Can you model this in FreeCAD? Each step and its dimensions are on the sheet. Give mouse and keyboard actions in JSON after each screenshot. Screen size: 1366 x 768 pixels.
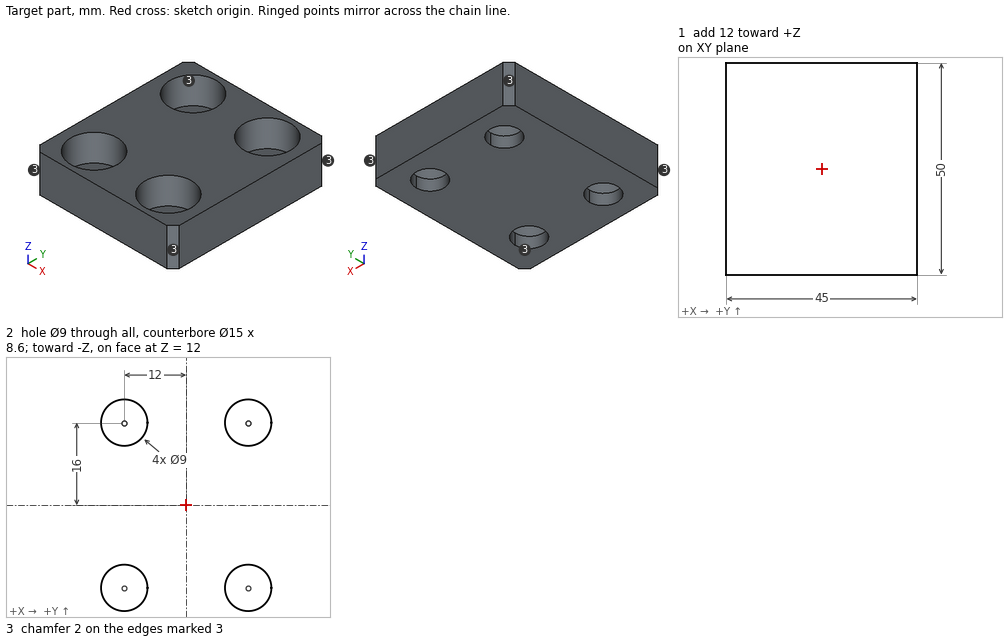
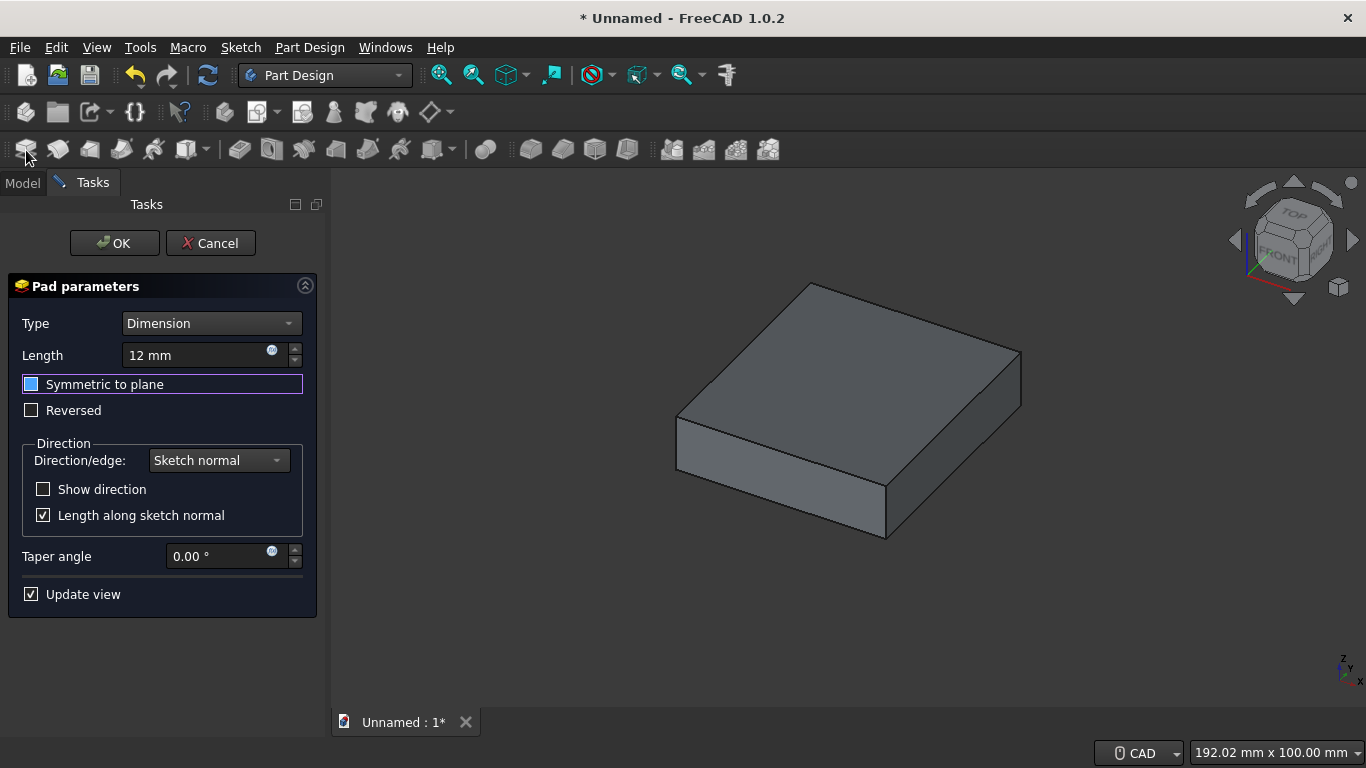
{"action": "left_click", "coordinate": [115, 243]}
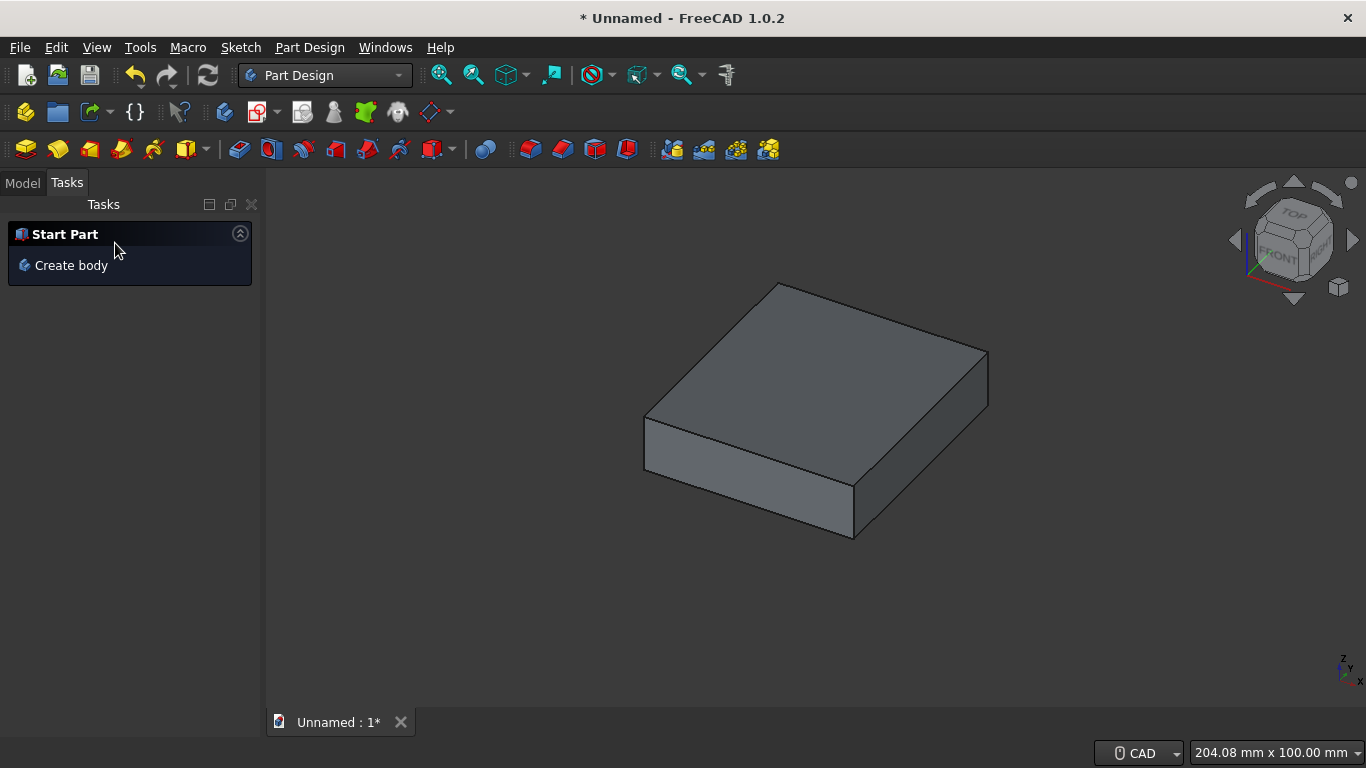
{"action": "left_click", "coordinate": [816, 384]}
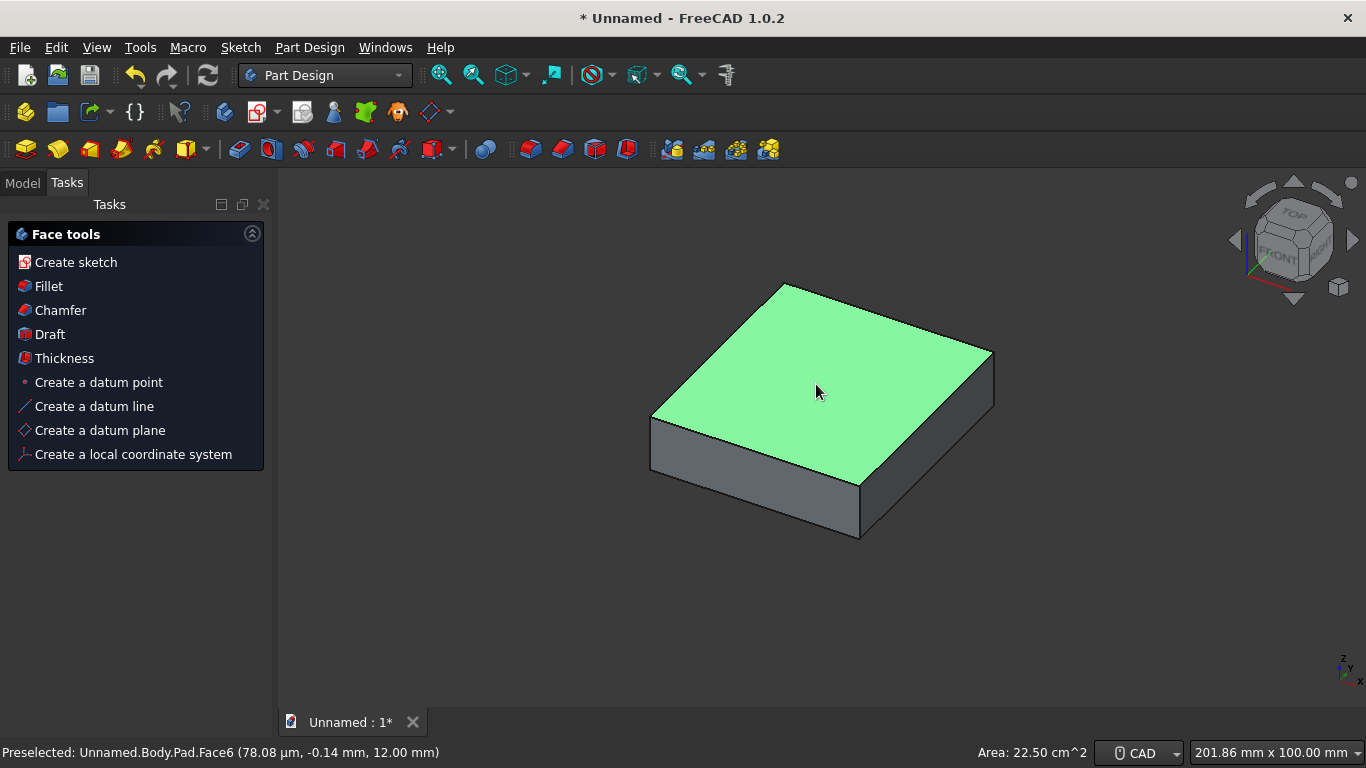
{"action": "left_click", "coordinate": [258, 112]}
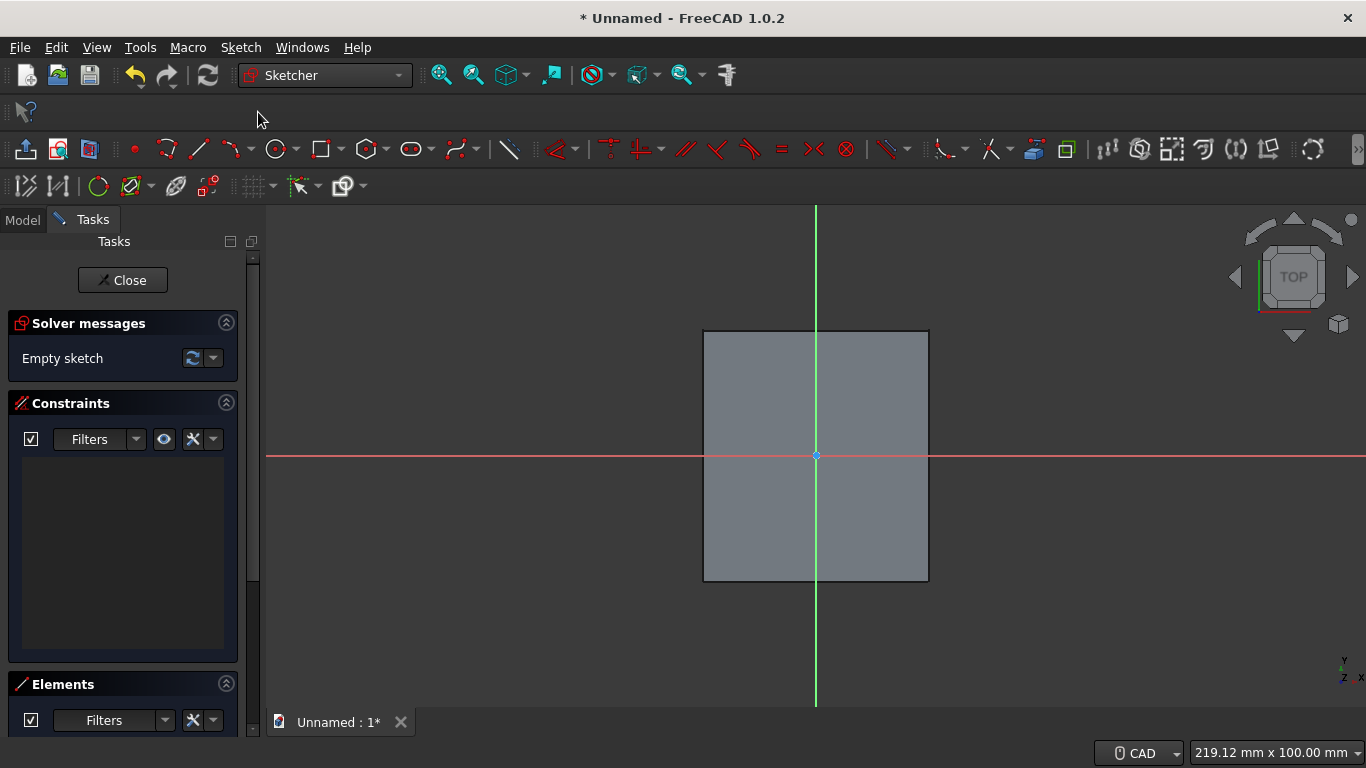
{"action": "scroll", "coordinate": [955, 456], "scroll_direction": "up", "scroll_amount": 2}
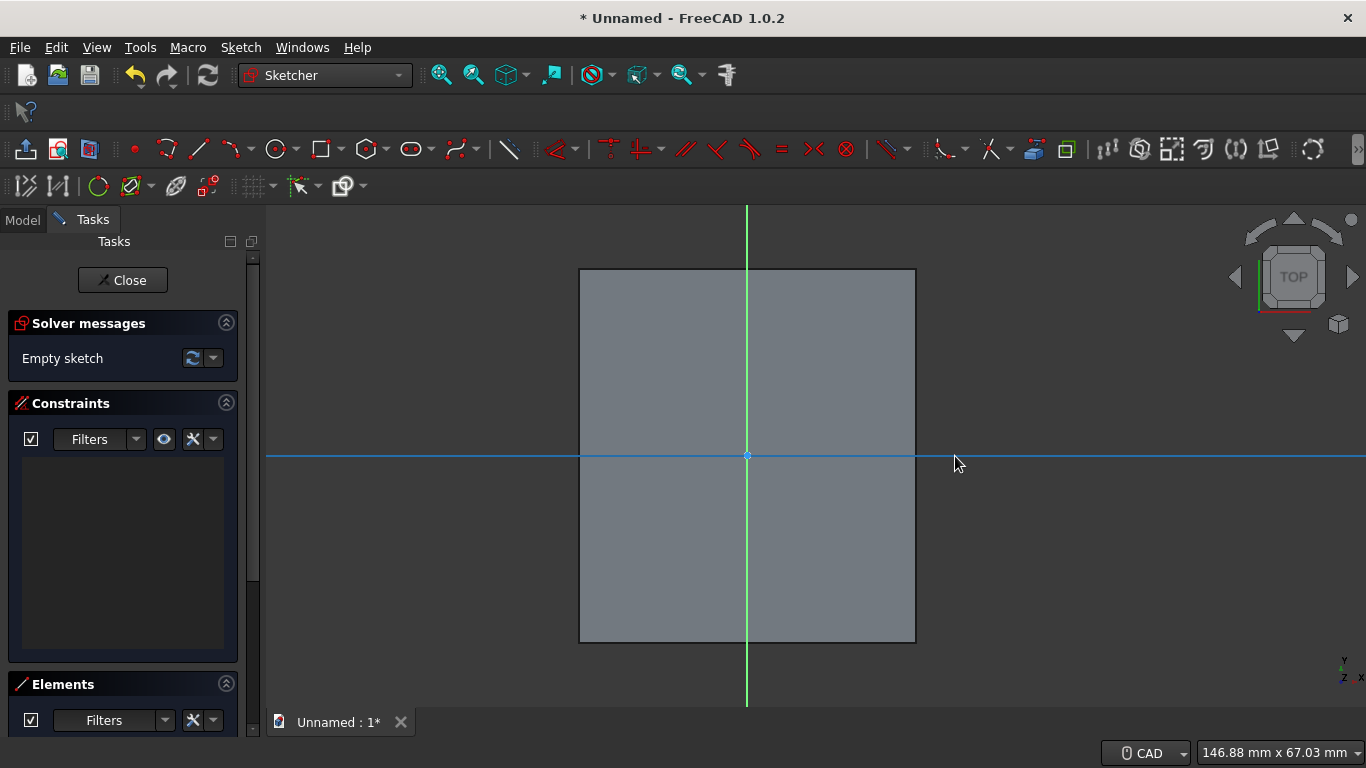
{"action": "left_click", "coordinate": [276, 150]}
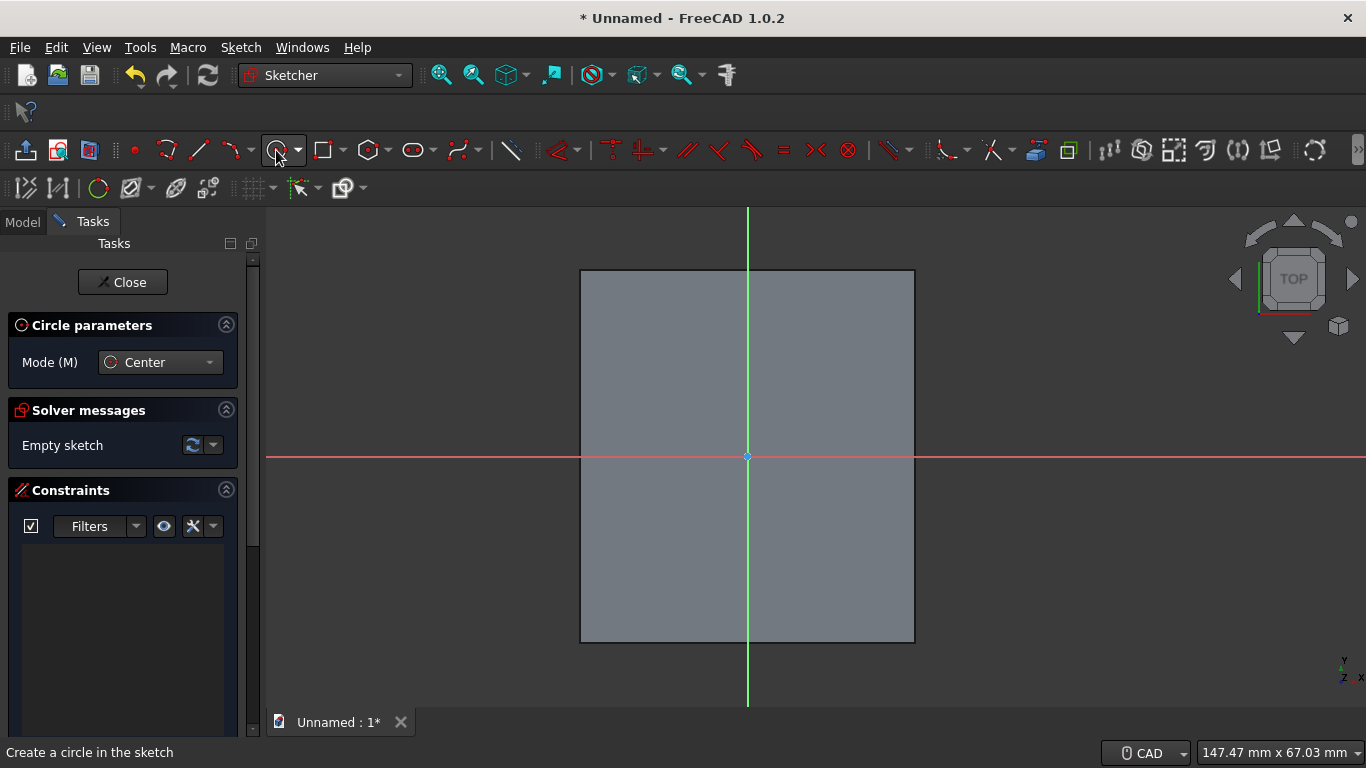
{"action": "left_click", "coordinate": [658, 337]}
{"action": "mouse_move", "coordinate": [682, 314]}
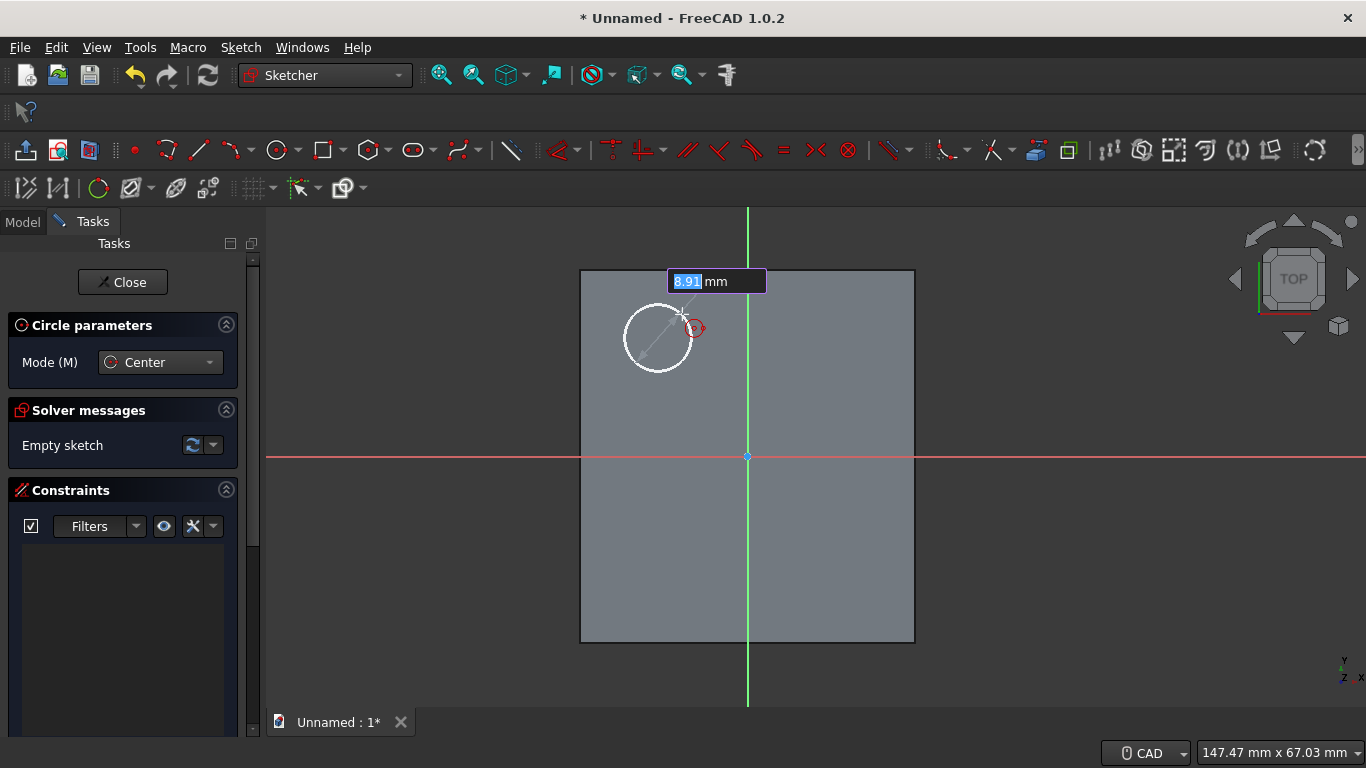
{"action": "type", "text": "9"}
{"action": "key", "text": "Return"}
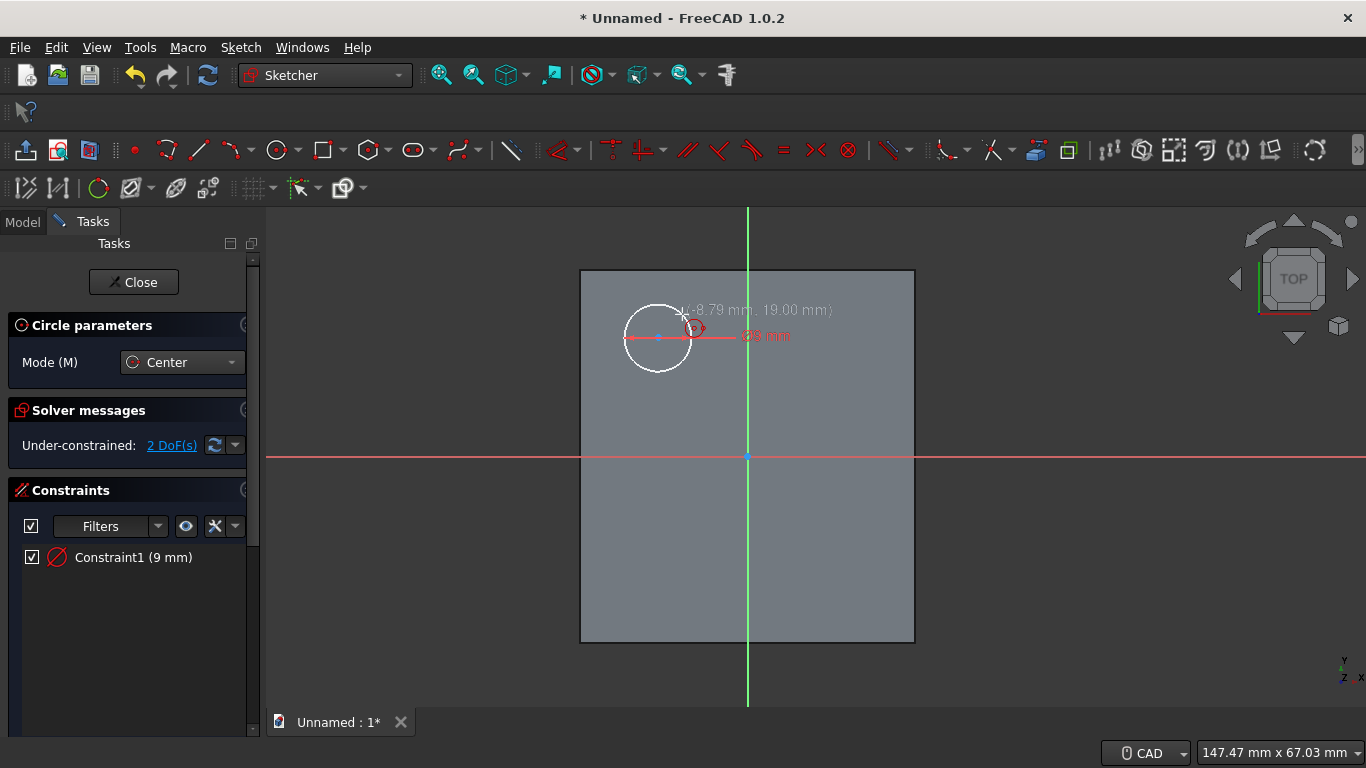
{"action": "left_click", "coordinate": [837, 337]}
{"action": "mouse_move", "coordinate": [861, 314]}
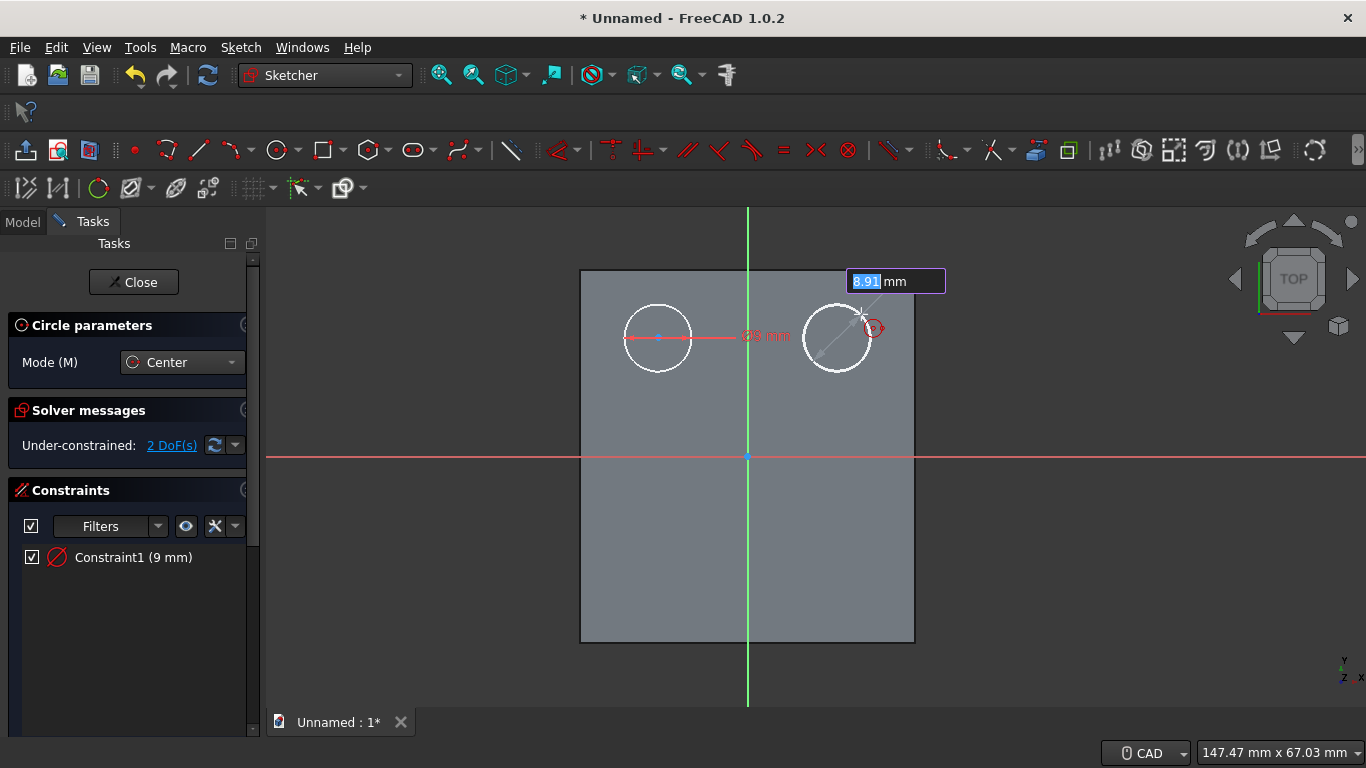
{"action": "type", "text": "9"}
{"action": "key", "text": "Return"}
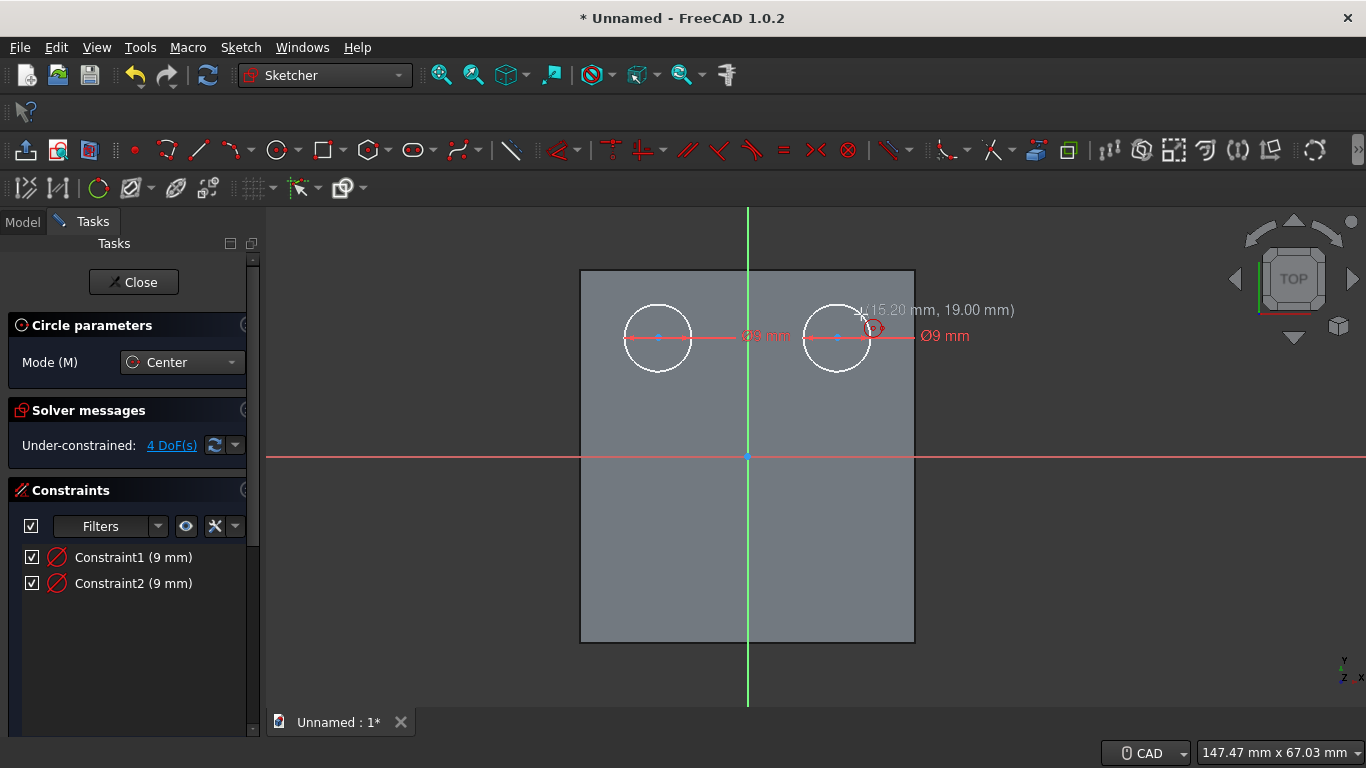
{"action": "left_click", "coordinate": [837, 576]}
{"action": "mouse_move", "coordinate": [861, 552]}